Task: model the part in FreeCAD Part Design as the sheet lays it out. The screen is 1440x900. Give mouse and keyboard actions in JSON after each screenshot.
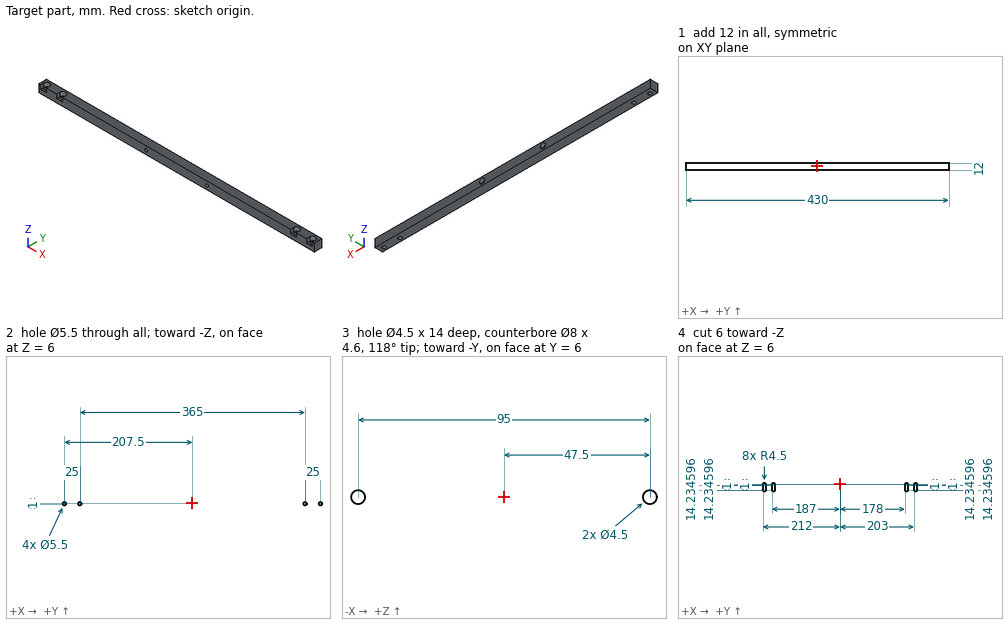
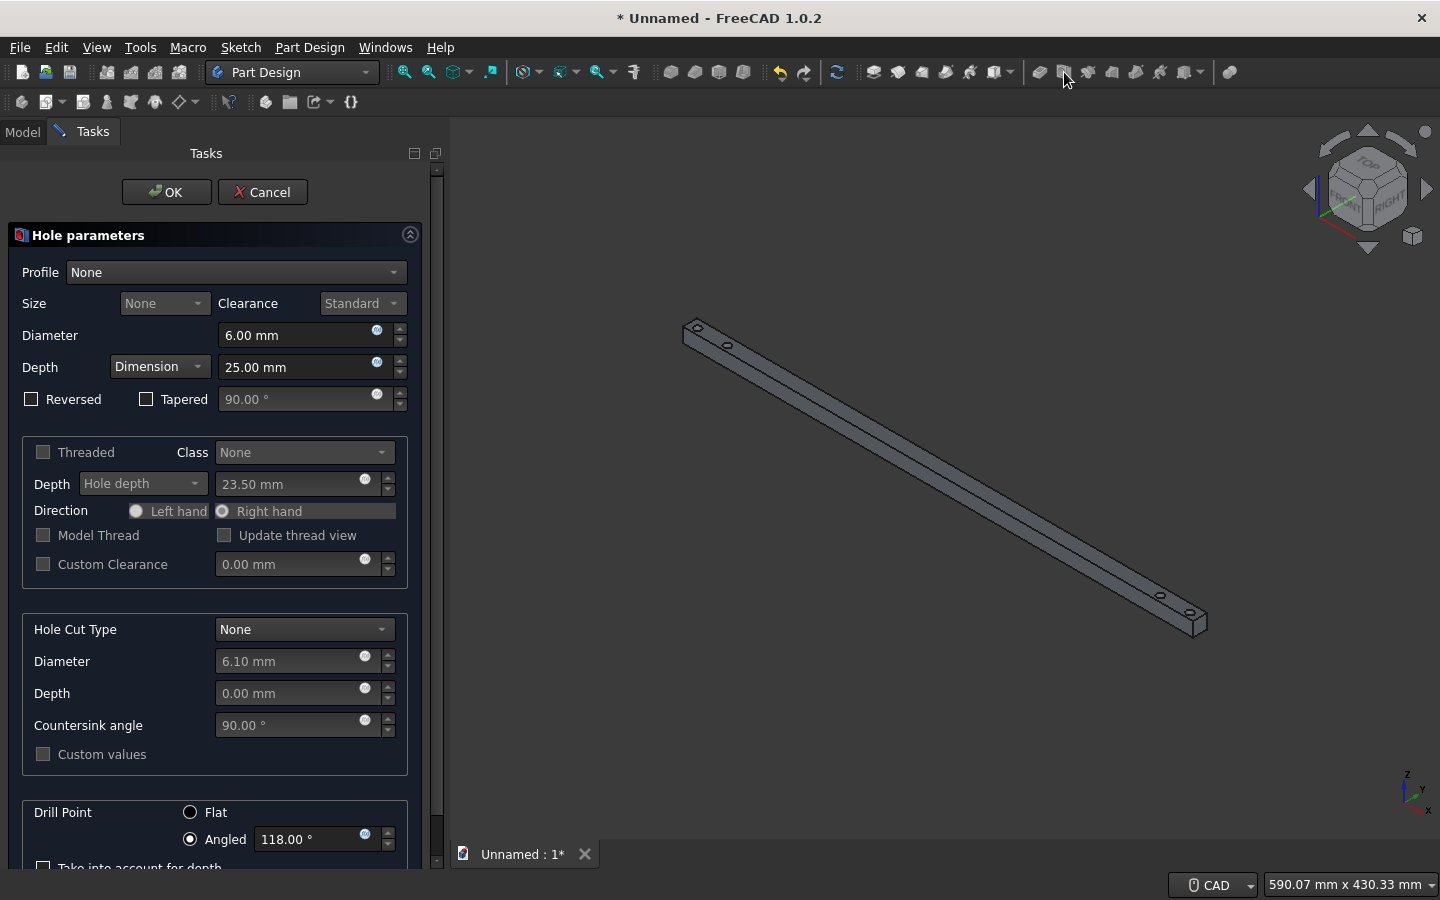
{"action": "triple_click", "coordinate": [305, 335]}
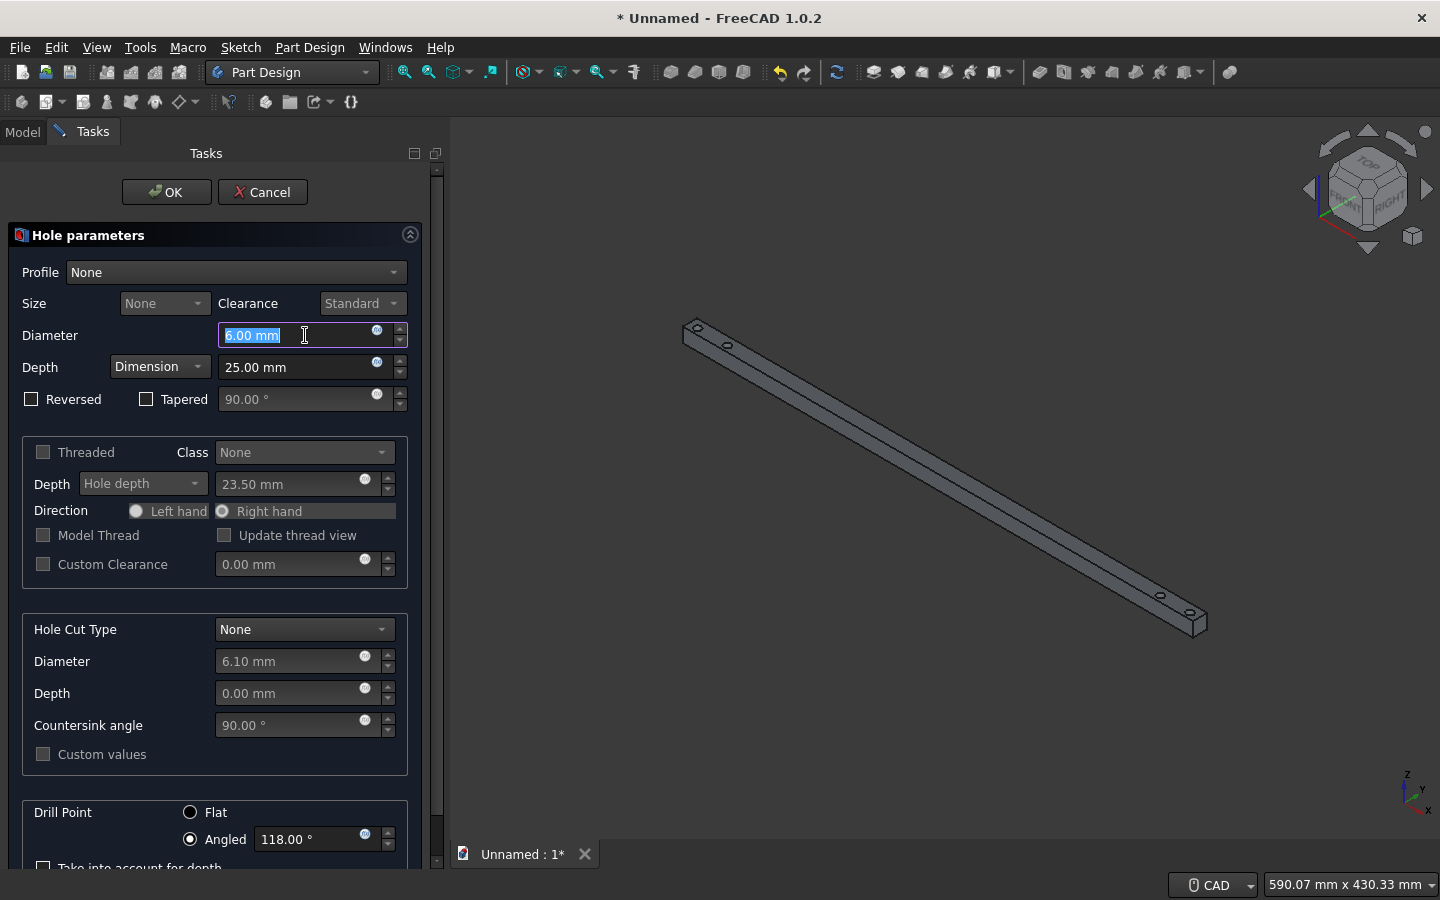
{"action": "type", "text": "5.5"}
{"action": "key", "text": "Tab"}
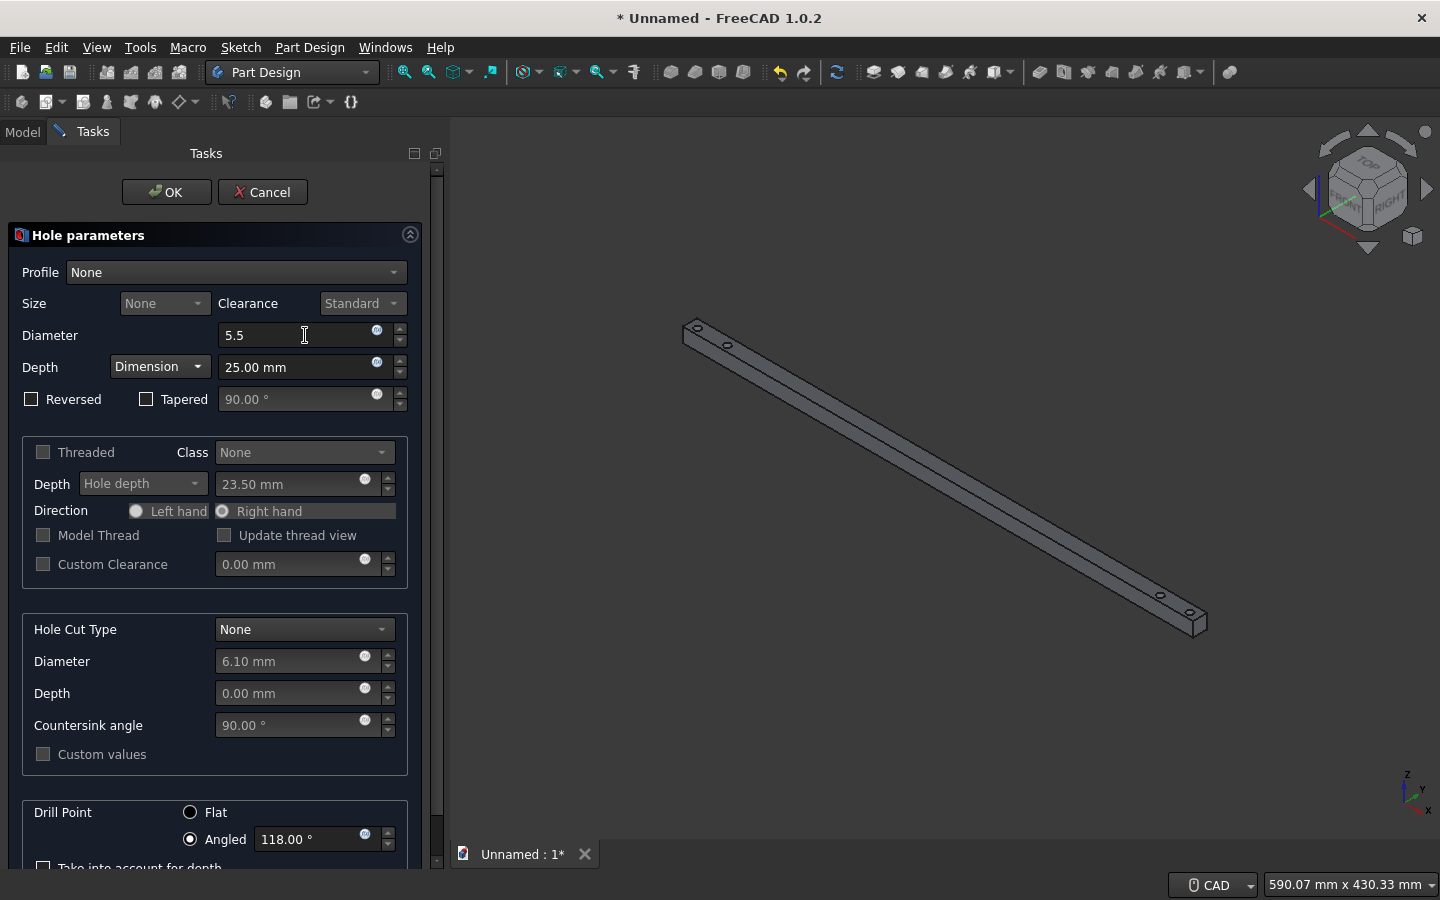
{"action": "left_click", "coordinate": [161, 366]}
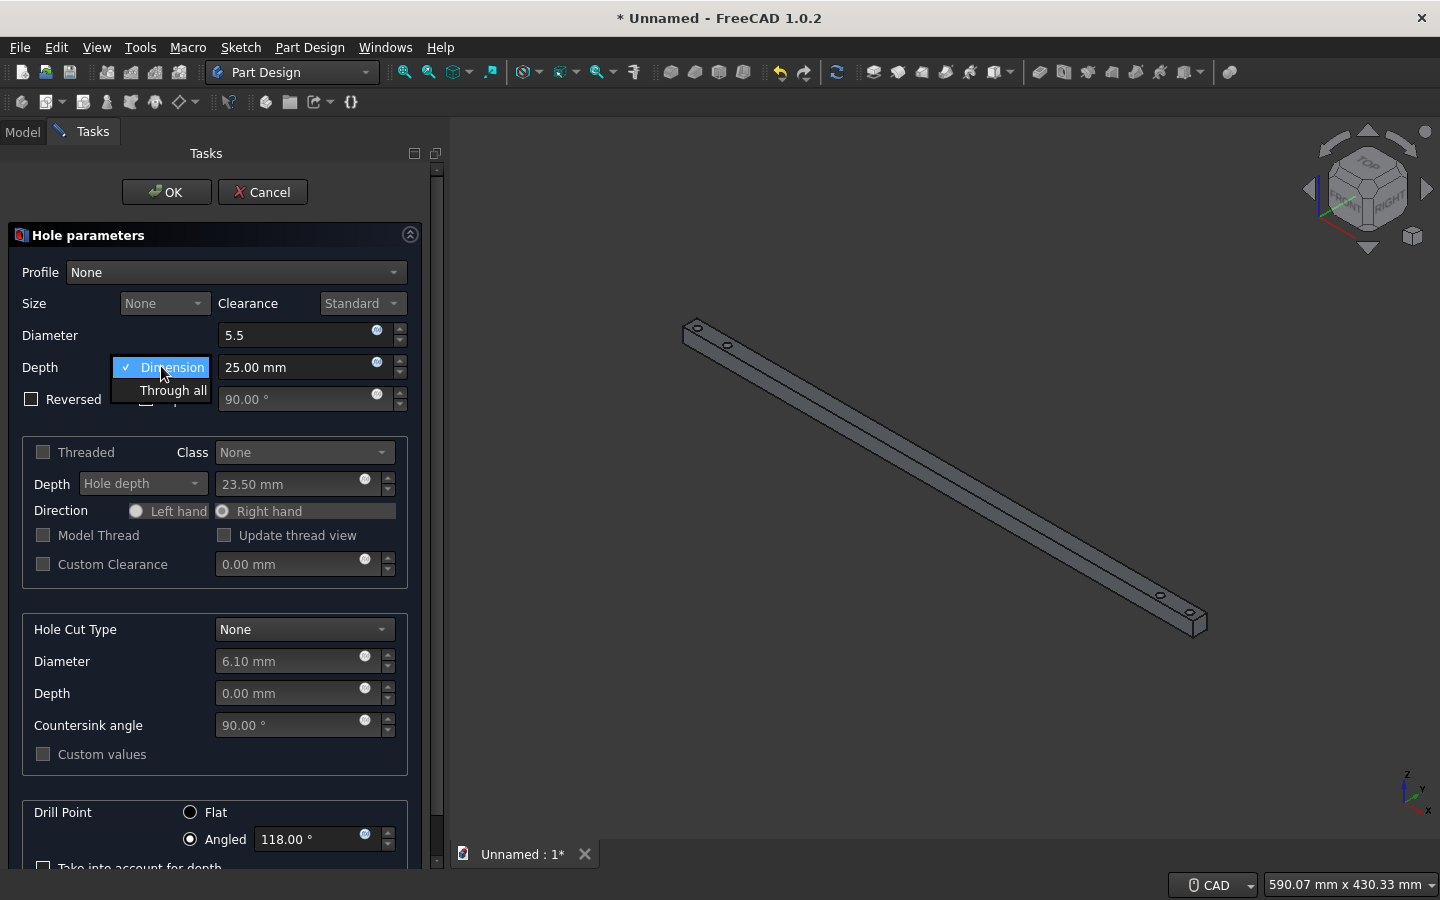
{"action": "left_click", "coordinate": [160, 390]}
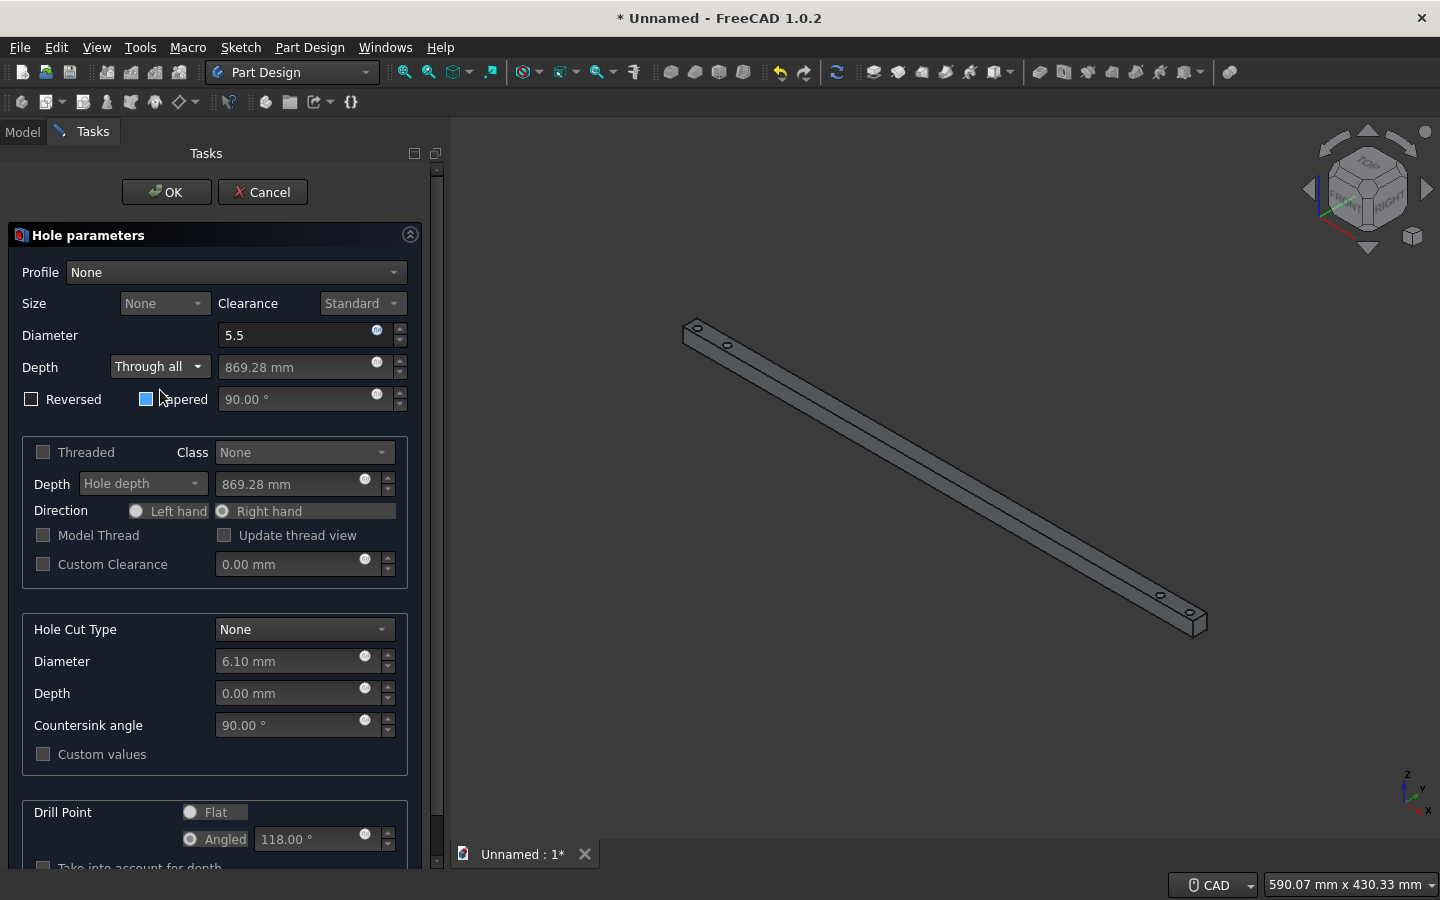
{"action": "left_click", "coordinate": [167, 192]}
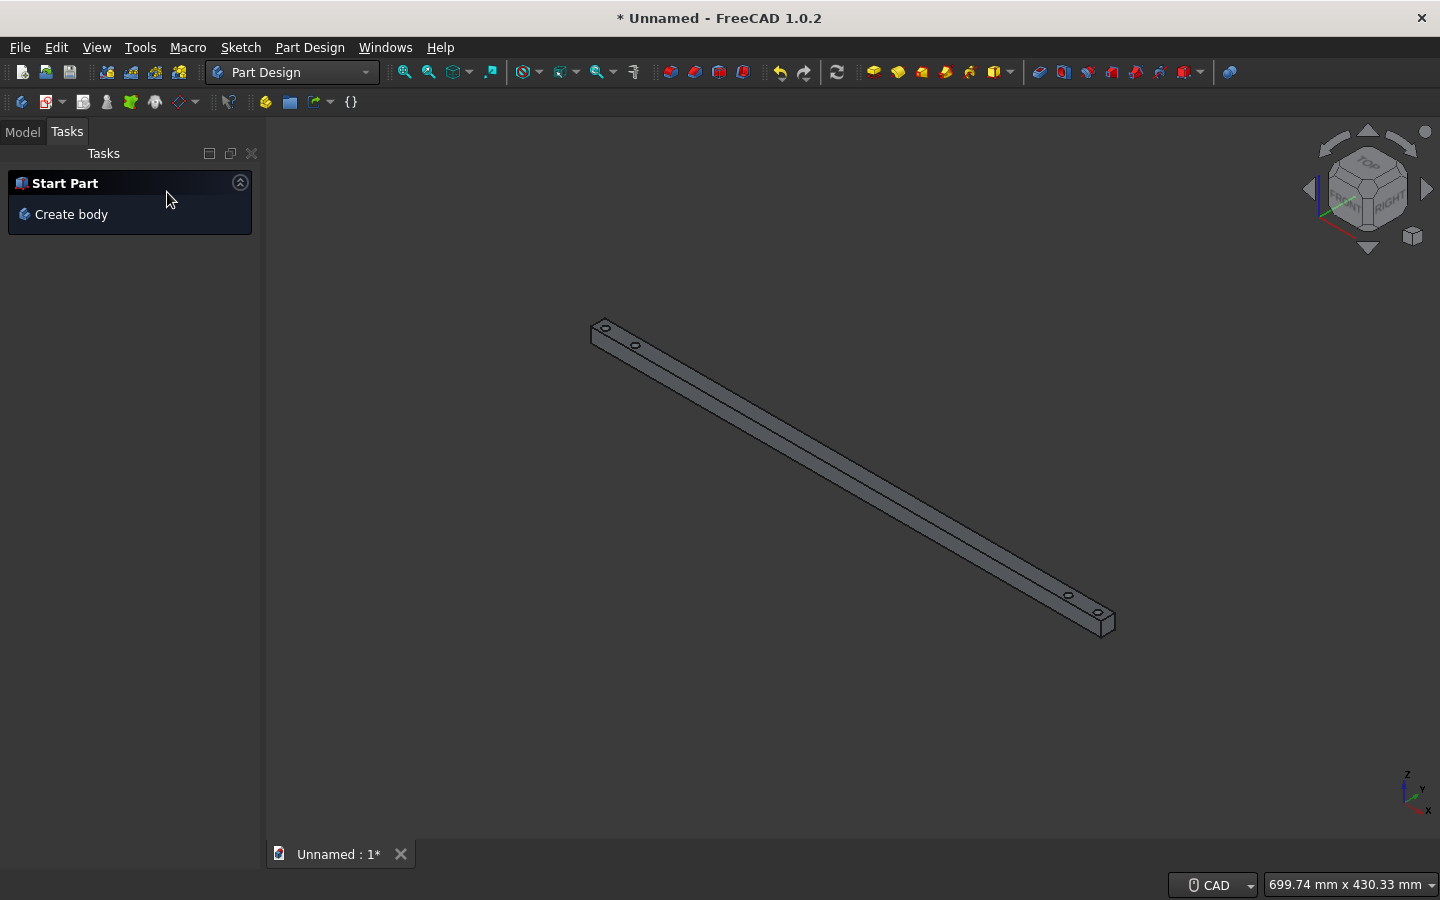
{"action": "left_click", "coordinate": [406, 72]}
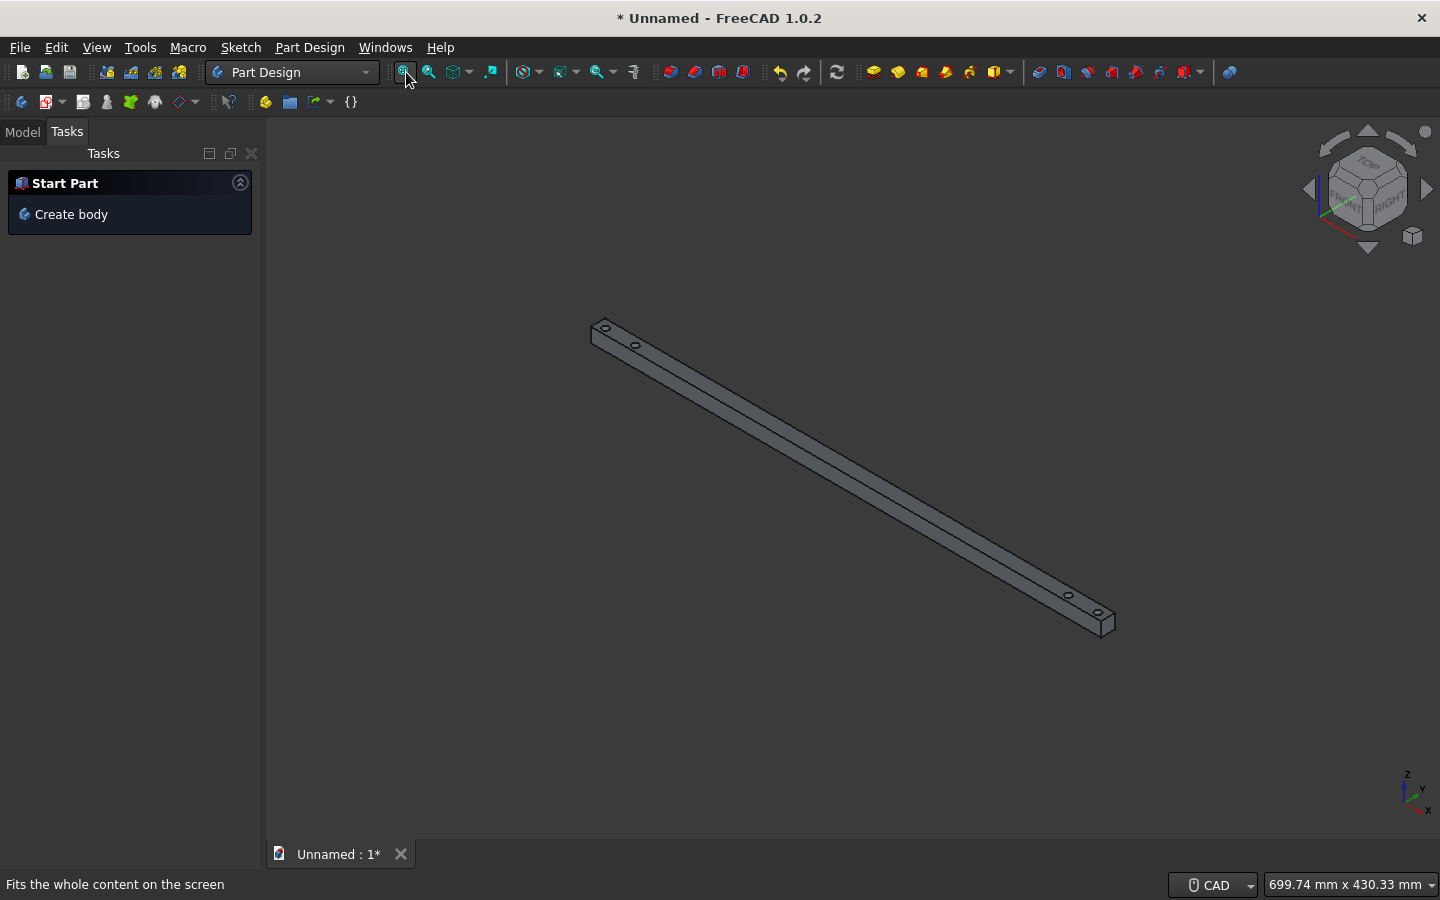
{"action": "key", "text": "4"}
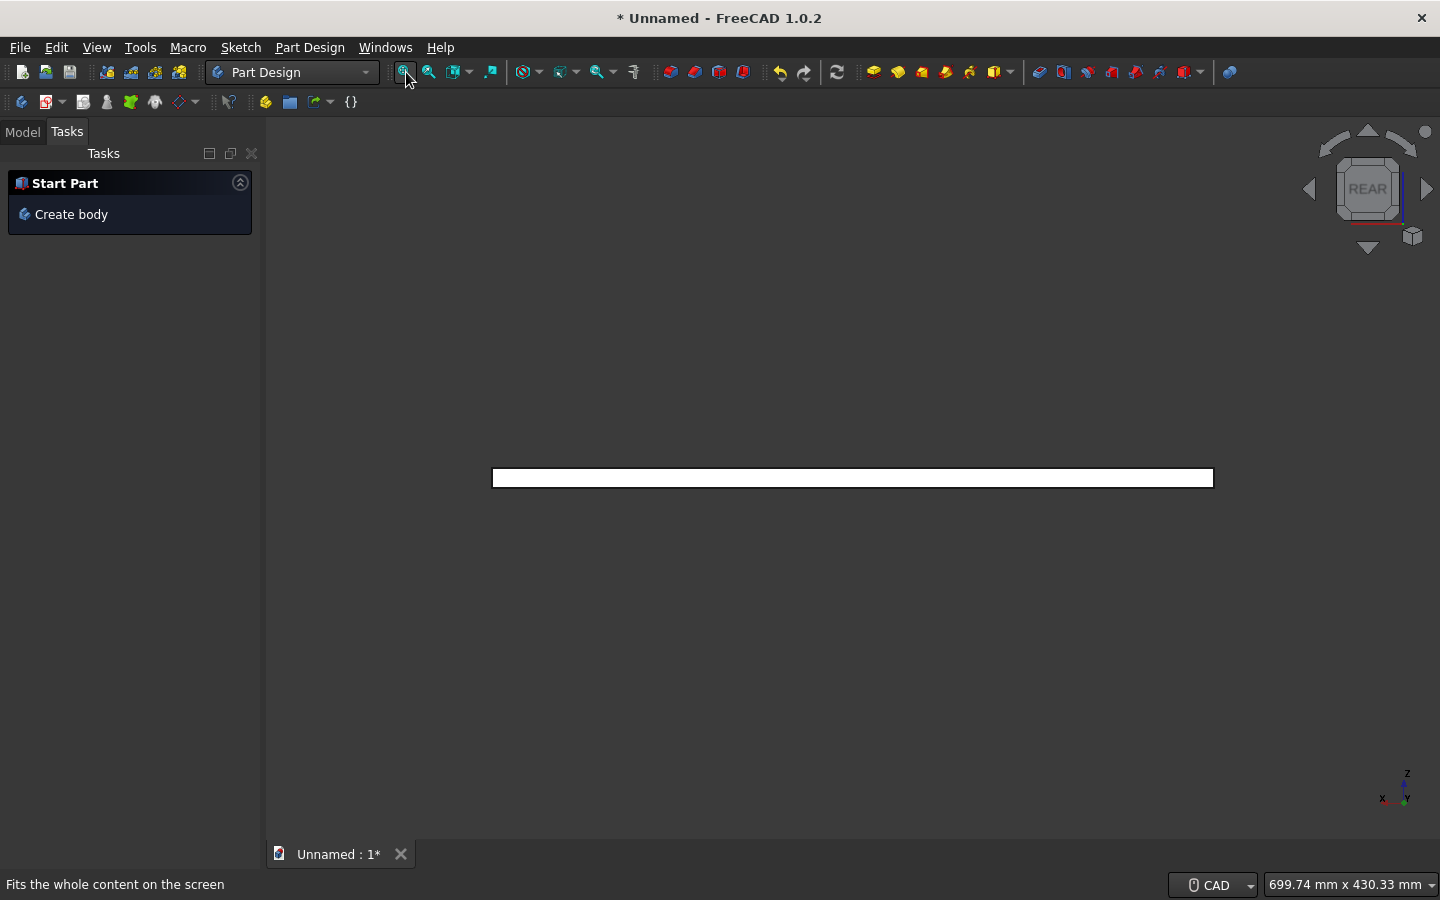
{"action": "left_click", "coordinate": [544, 477]}